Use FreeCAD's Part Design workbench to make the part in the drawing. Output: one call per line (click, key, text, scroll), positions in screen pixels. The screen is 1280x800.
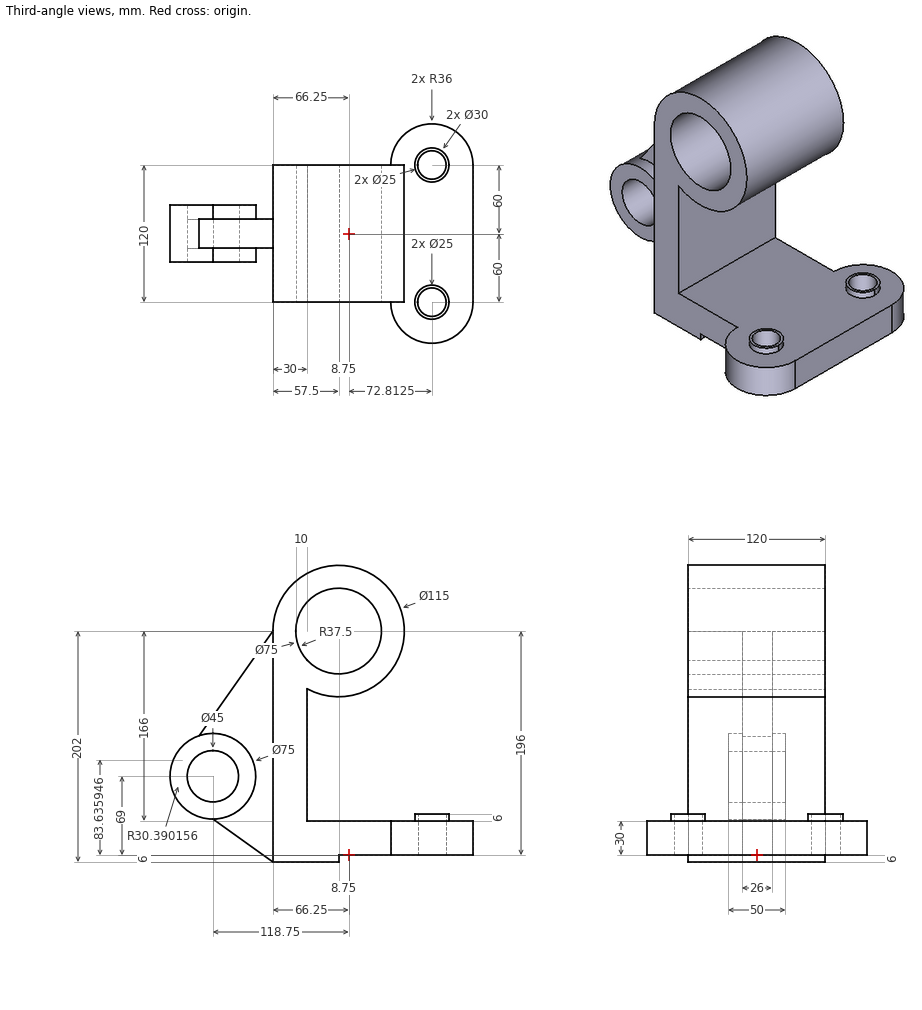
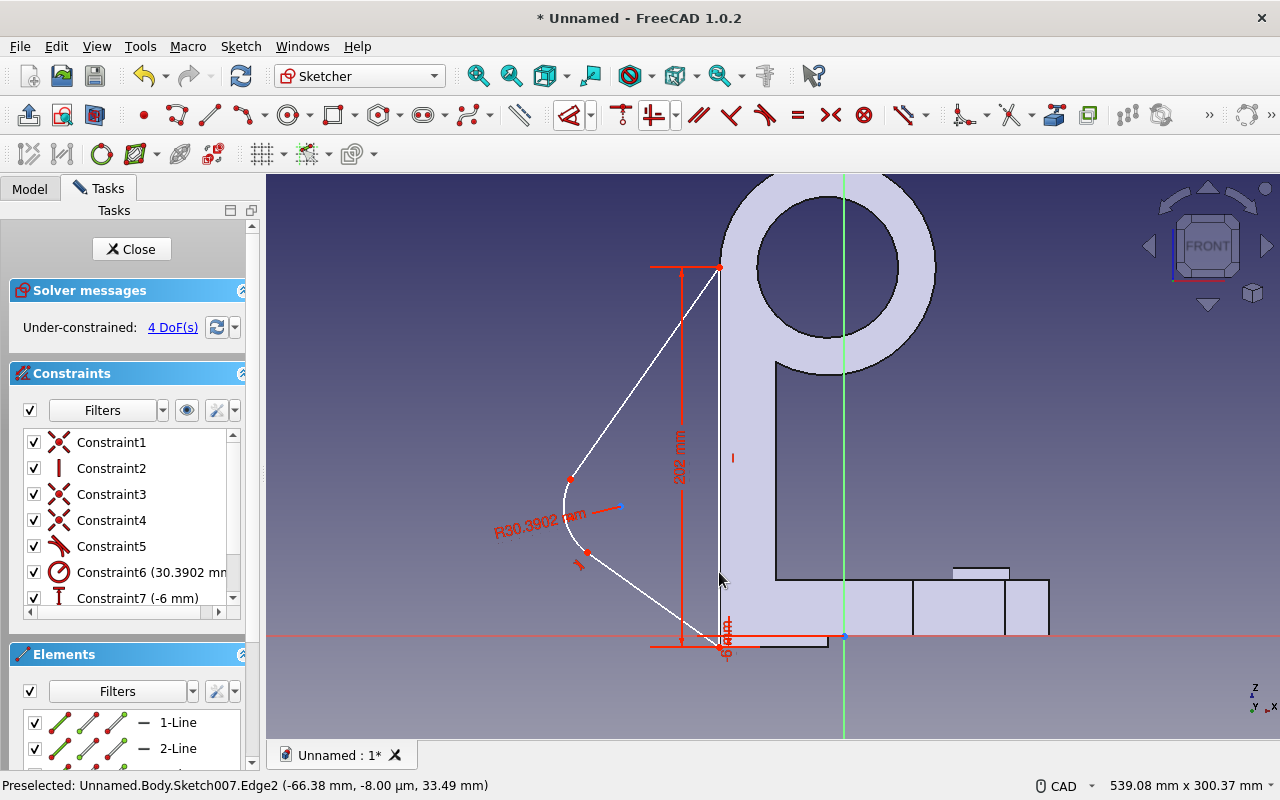
click(621, 507)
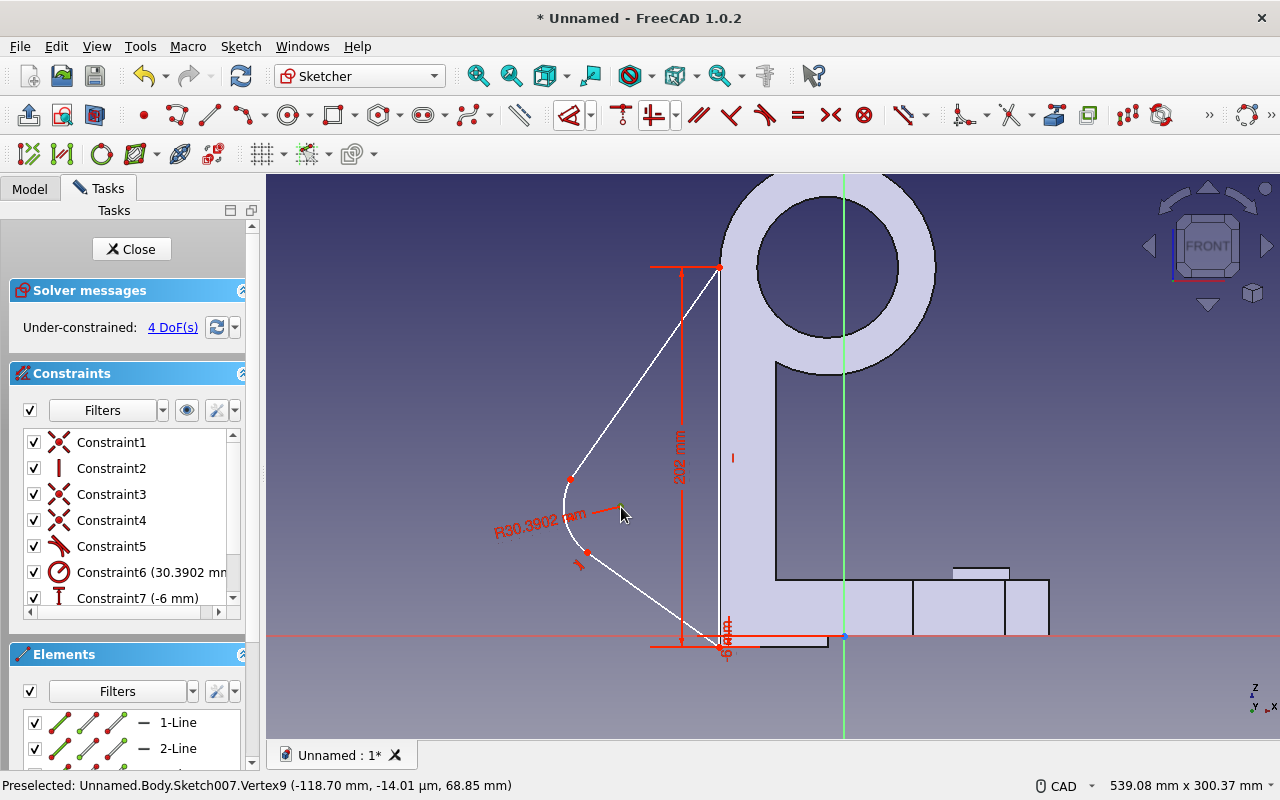
click(590, 116)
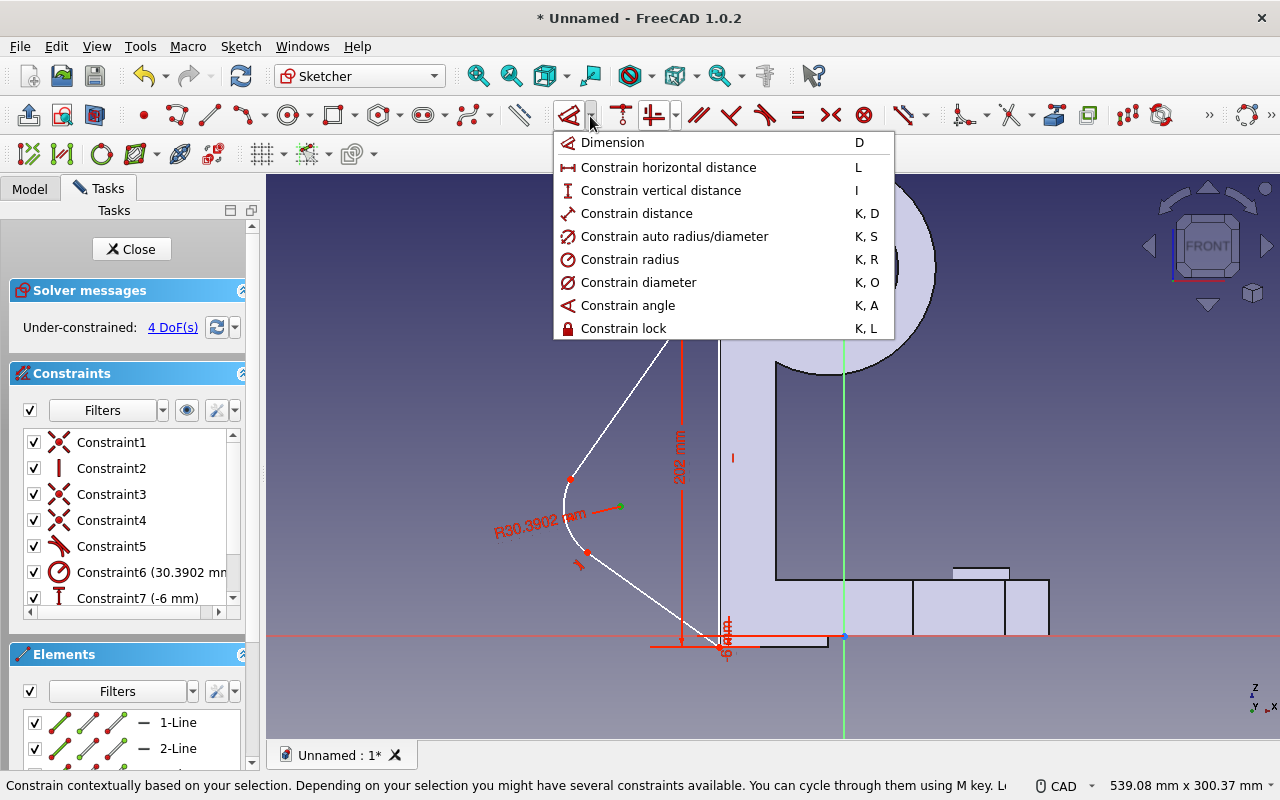
click(724, 190)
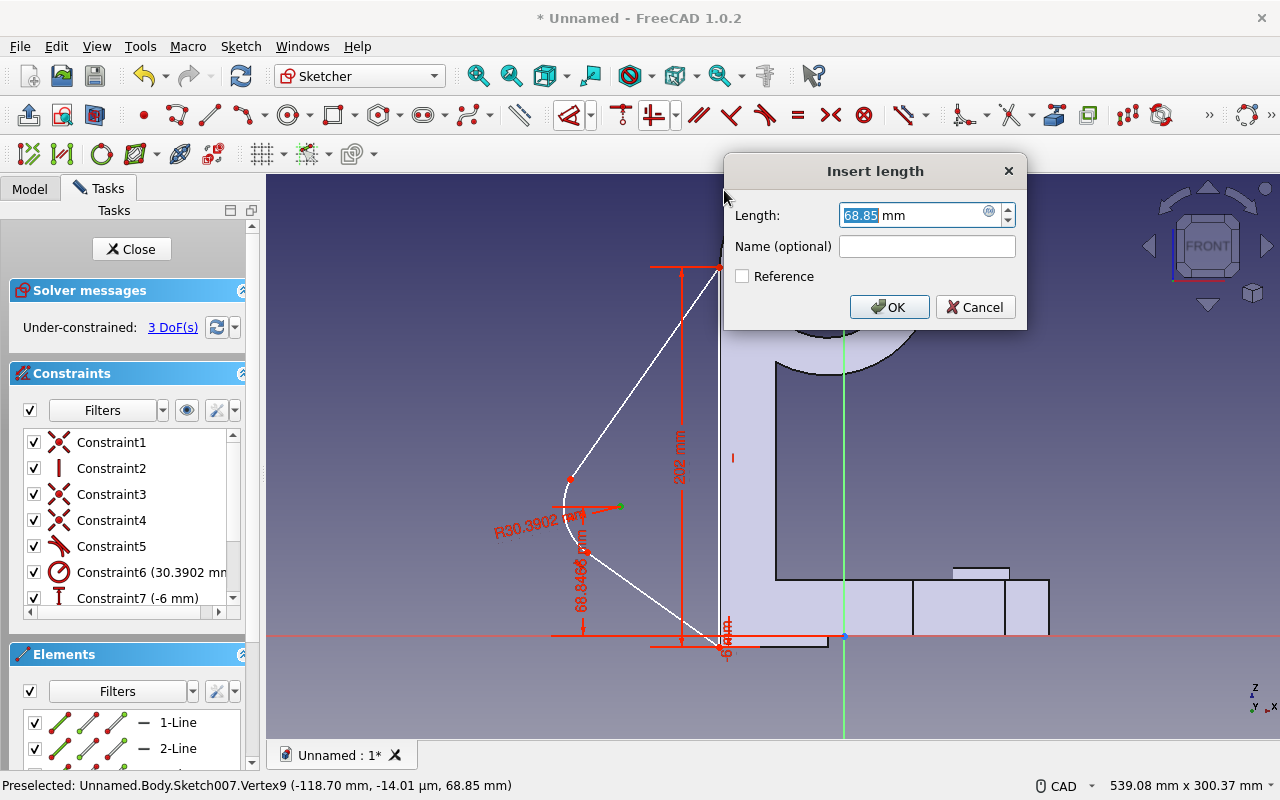
text(69)
key(Return)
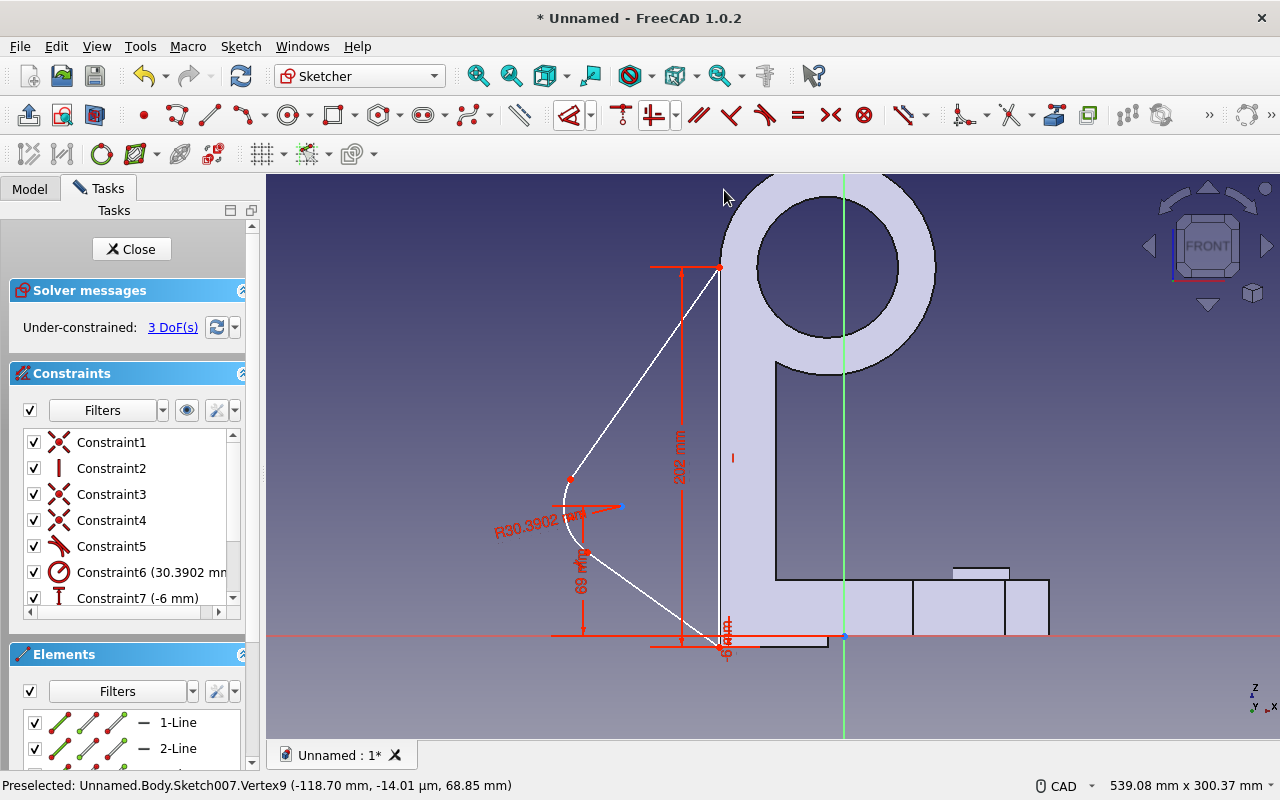
click(719, 267)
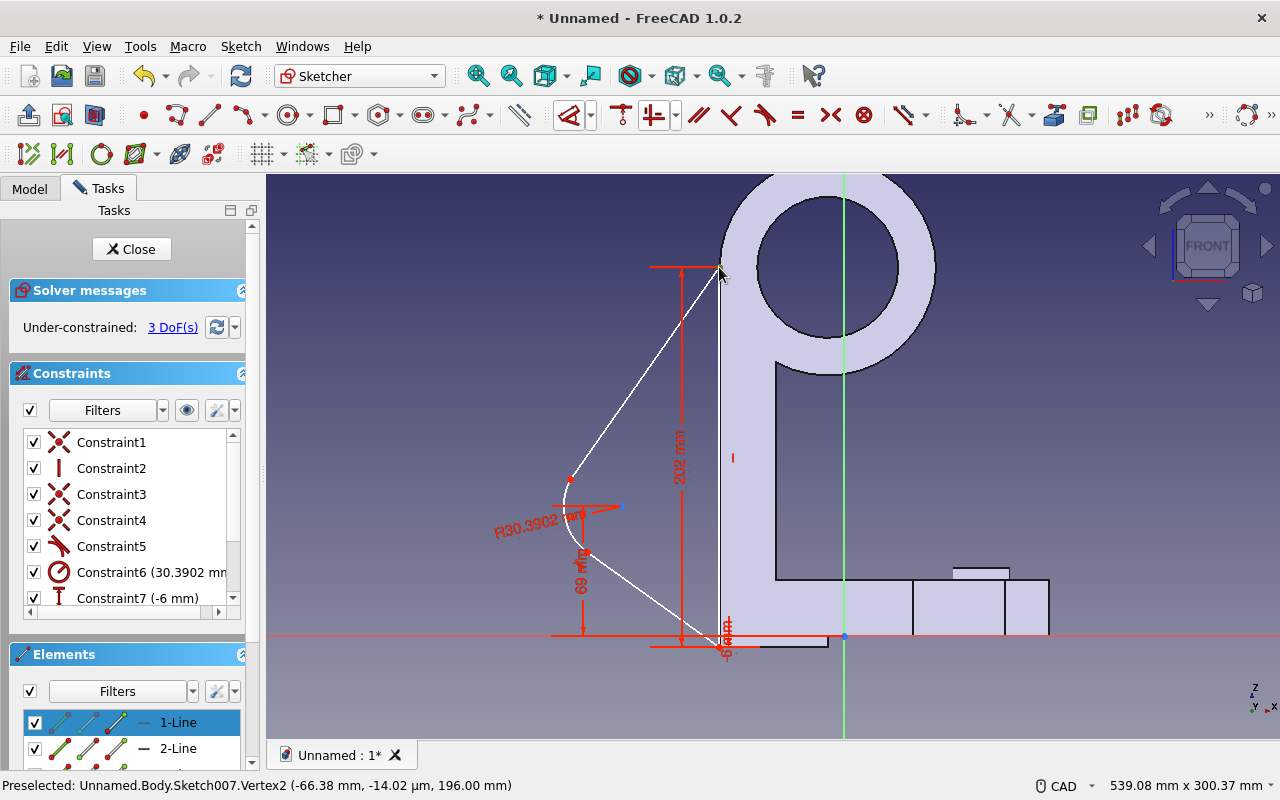
key(l)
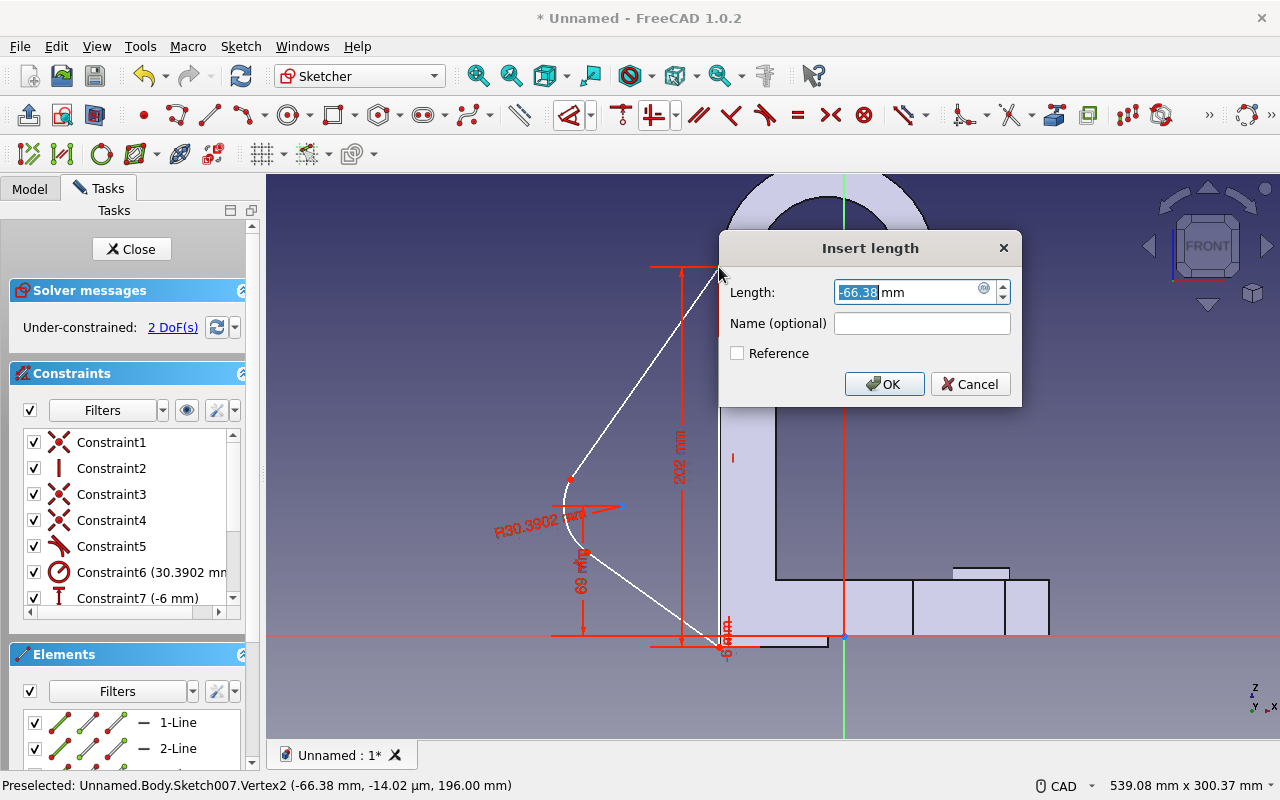
text(-66.25)
key(Return)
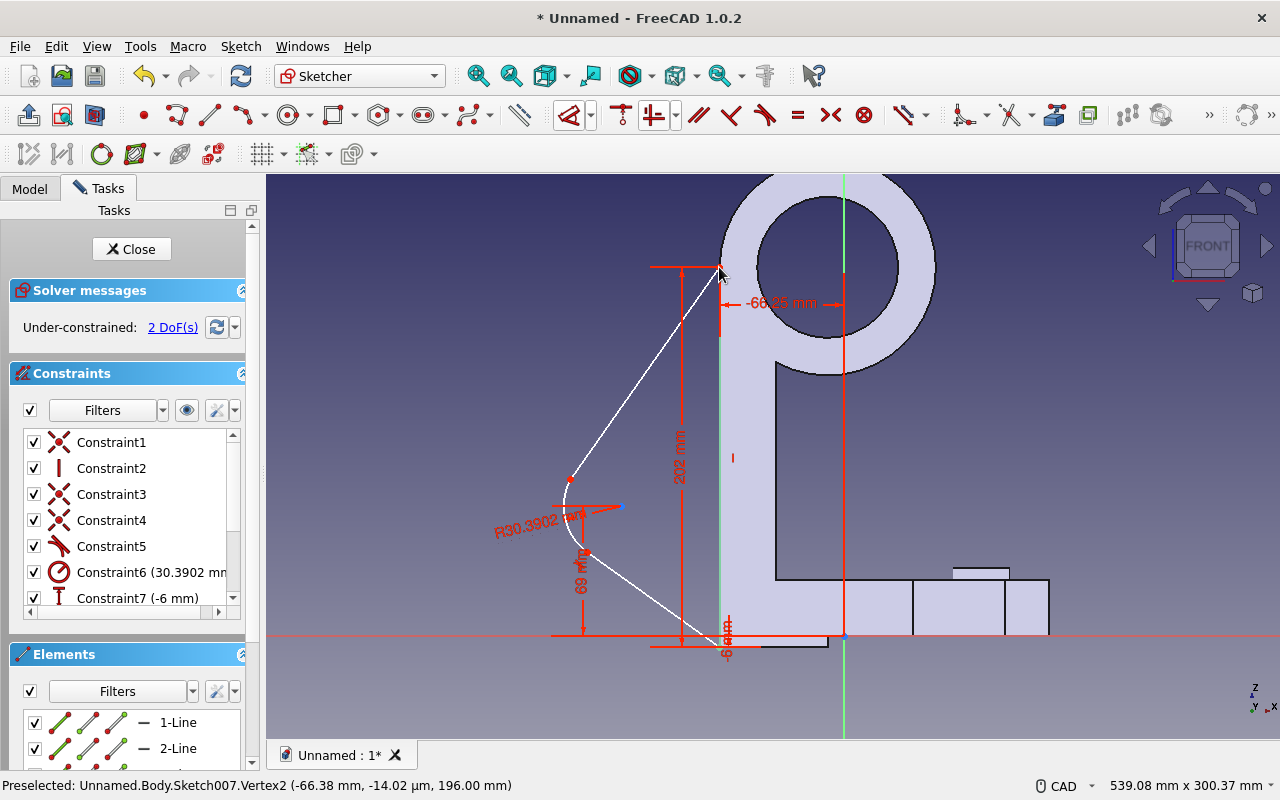
click(621, 506)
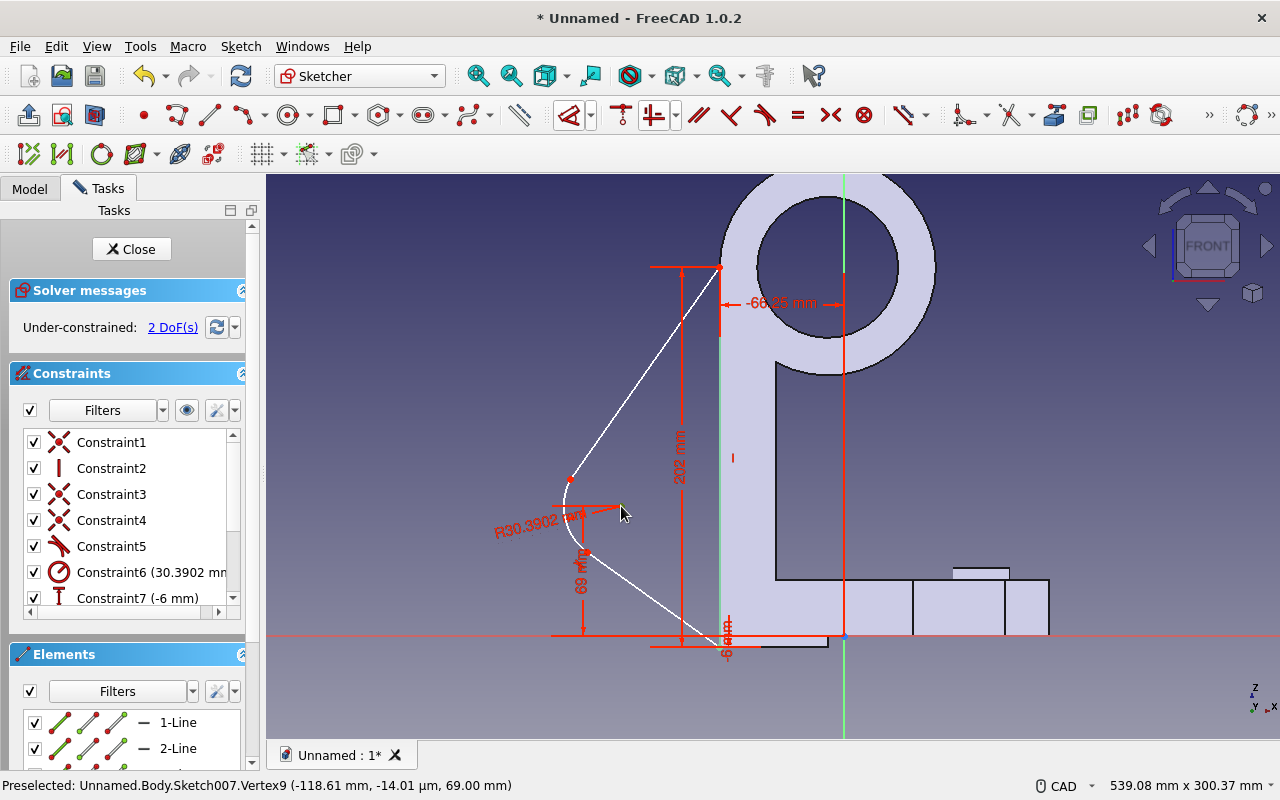
click(590, 116)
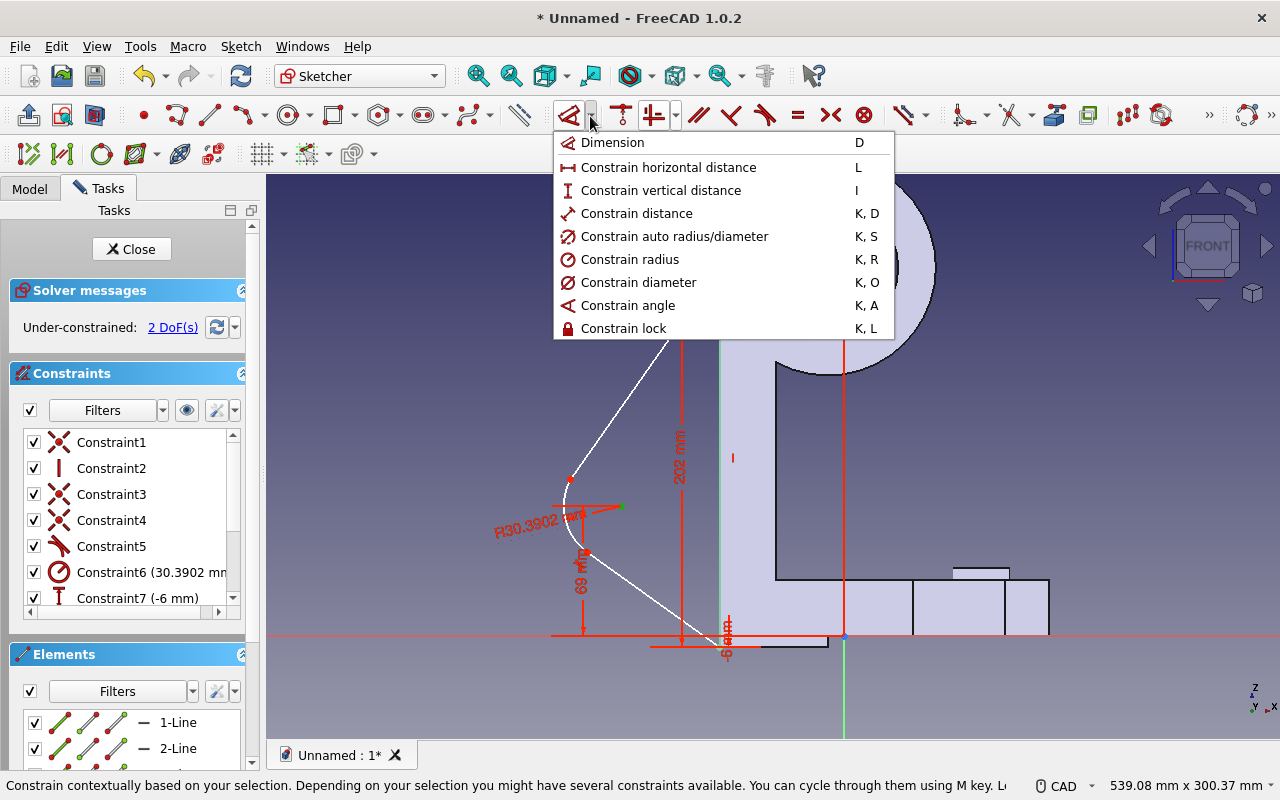
click(724, 168)